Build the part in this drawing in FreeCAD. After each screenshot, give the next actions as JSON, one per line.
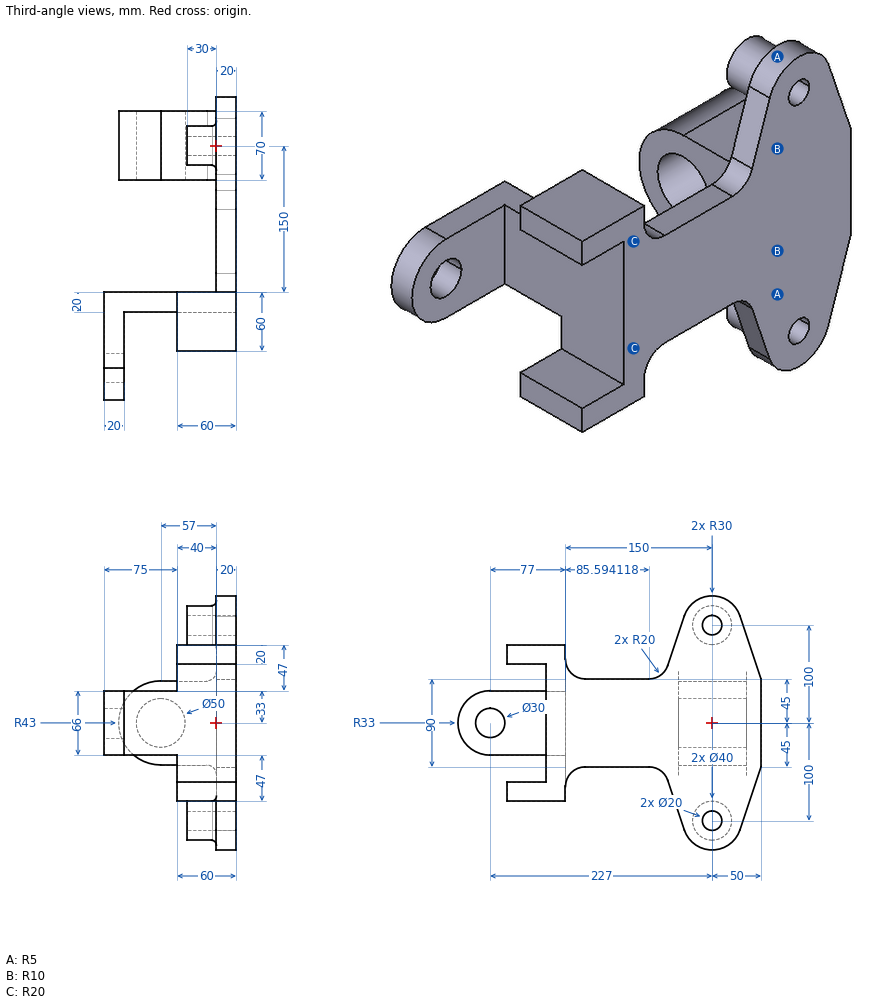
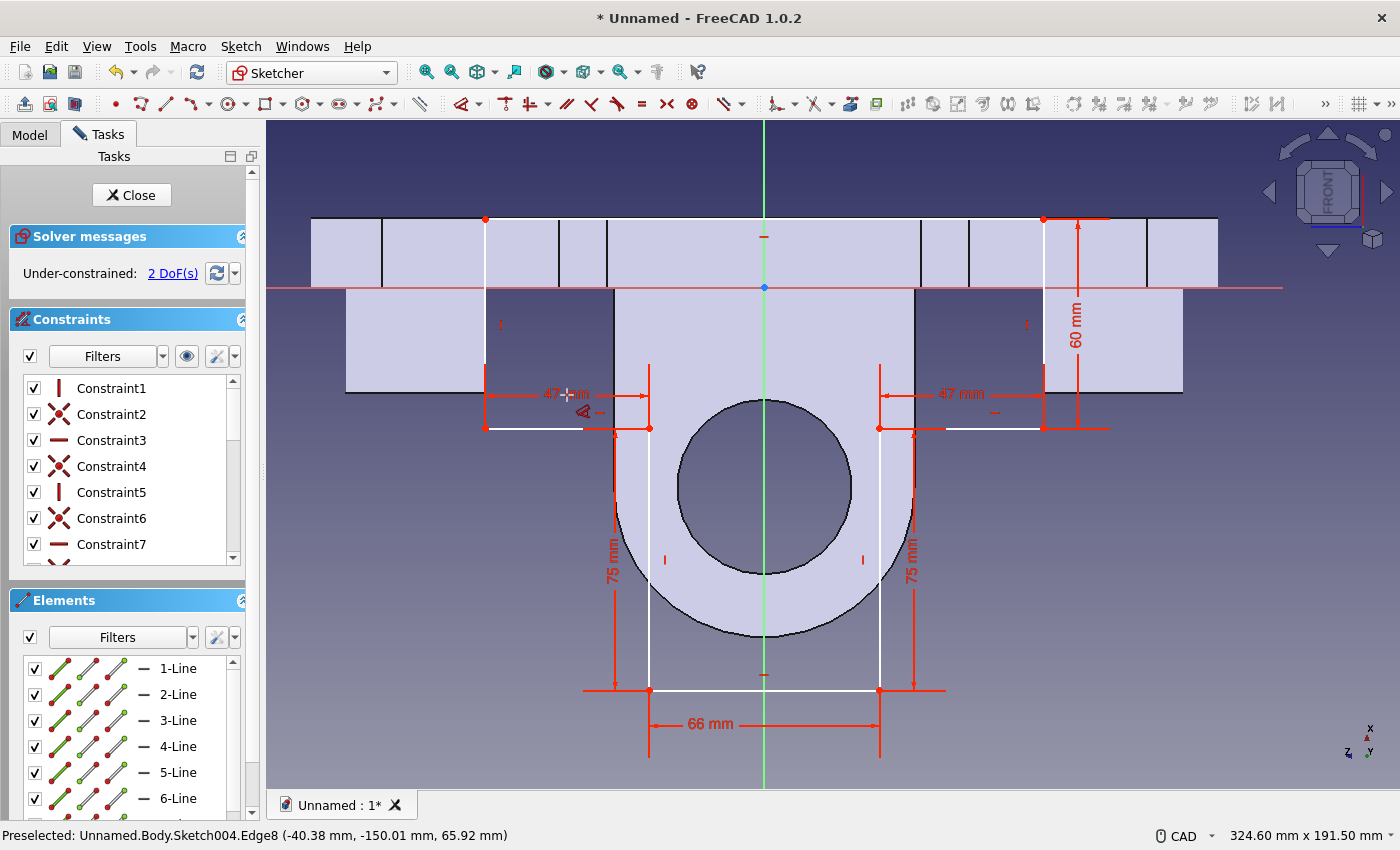
{"action": "left_click", "coordinate": [649, 429]}
{"action": "left_click", "coordinate": [707, 254]}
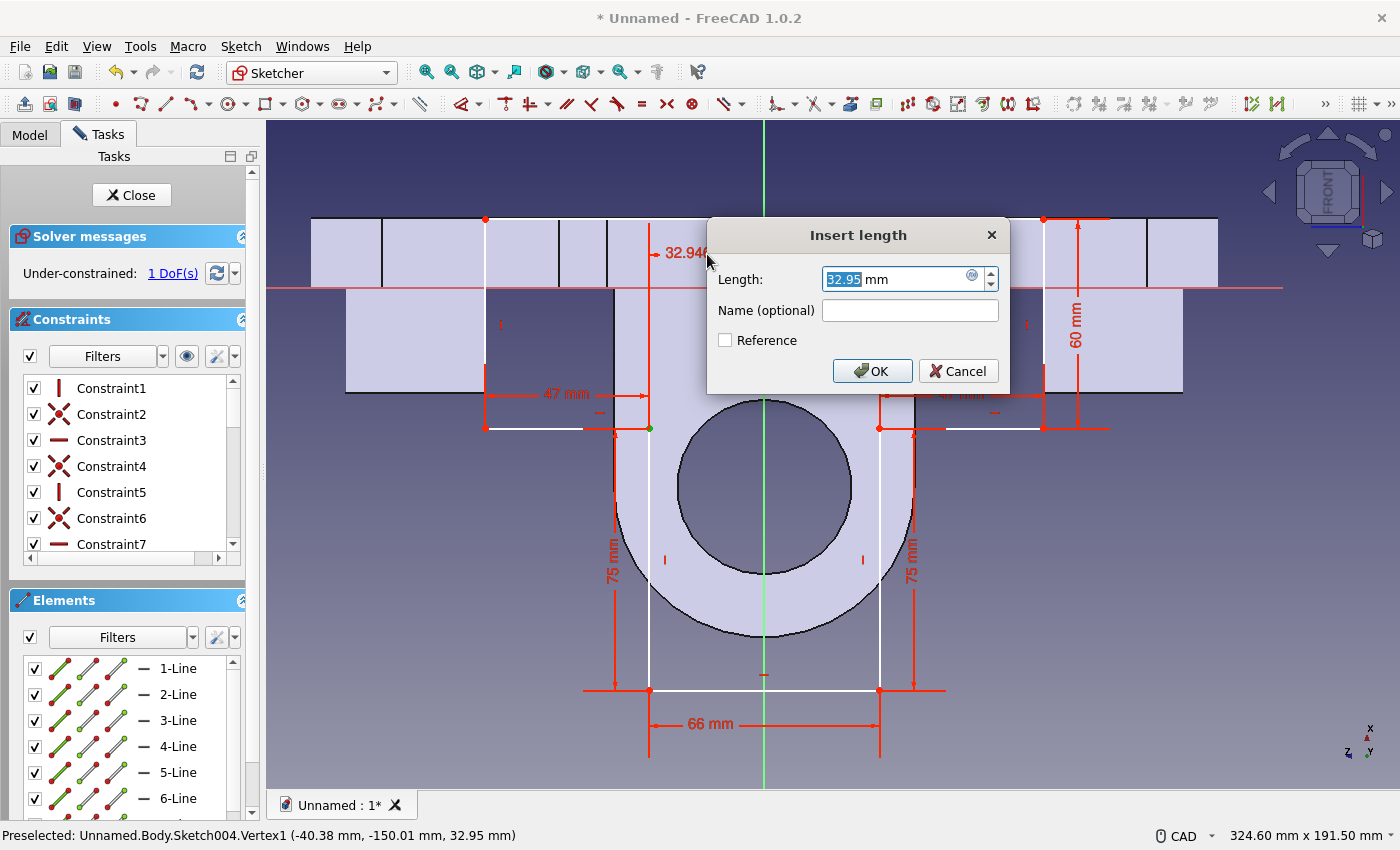
{"action": "type", "text": "33"}
{"action": "key", "text": "Return"}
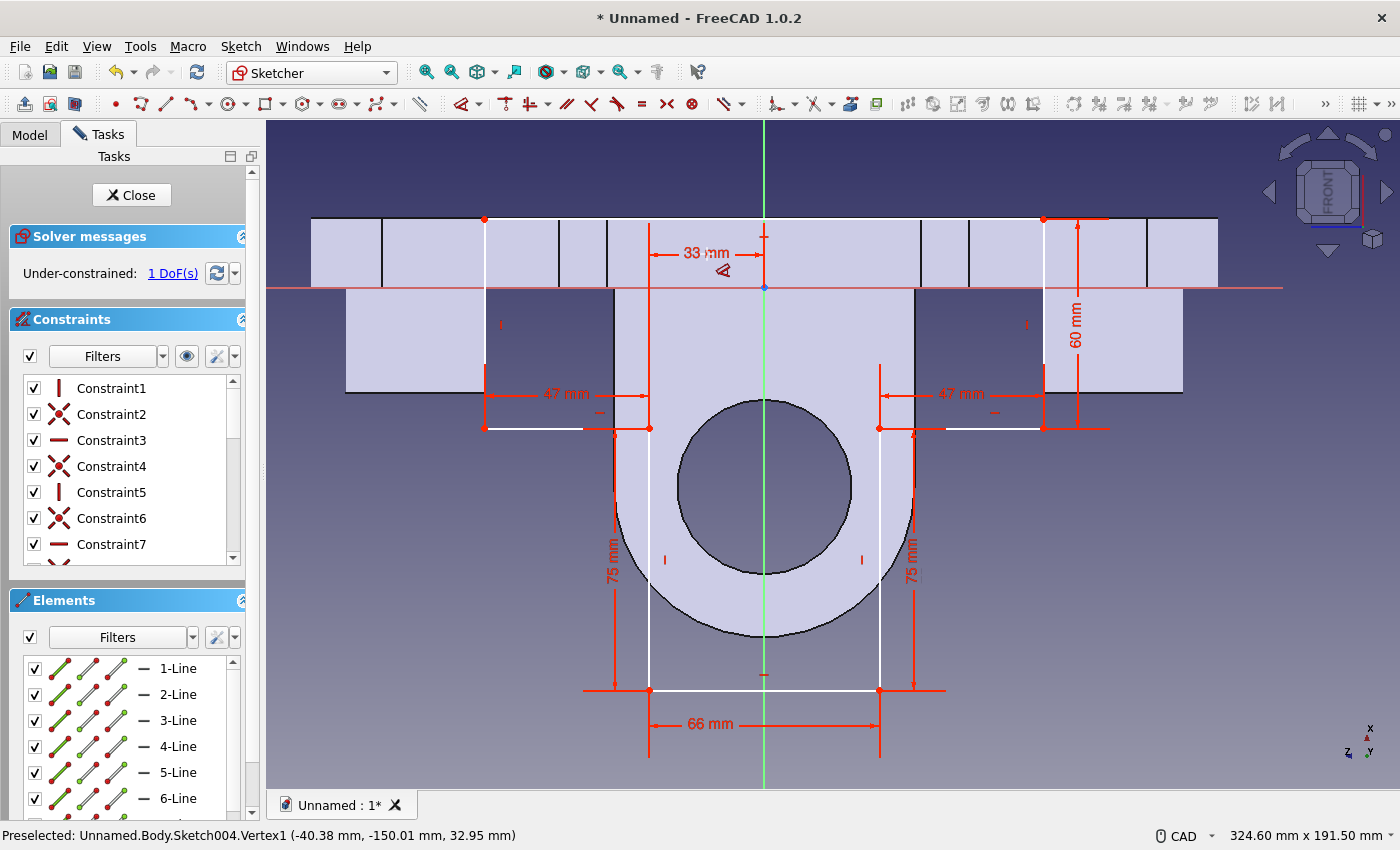
{"action": "left_click", "coordinate": [649, 429]}
{"action": "left_click", "coordinate": [615, 358]}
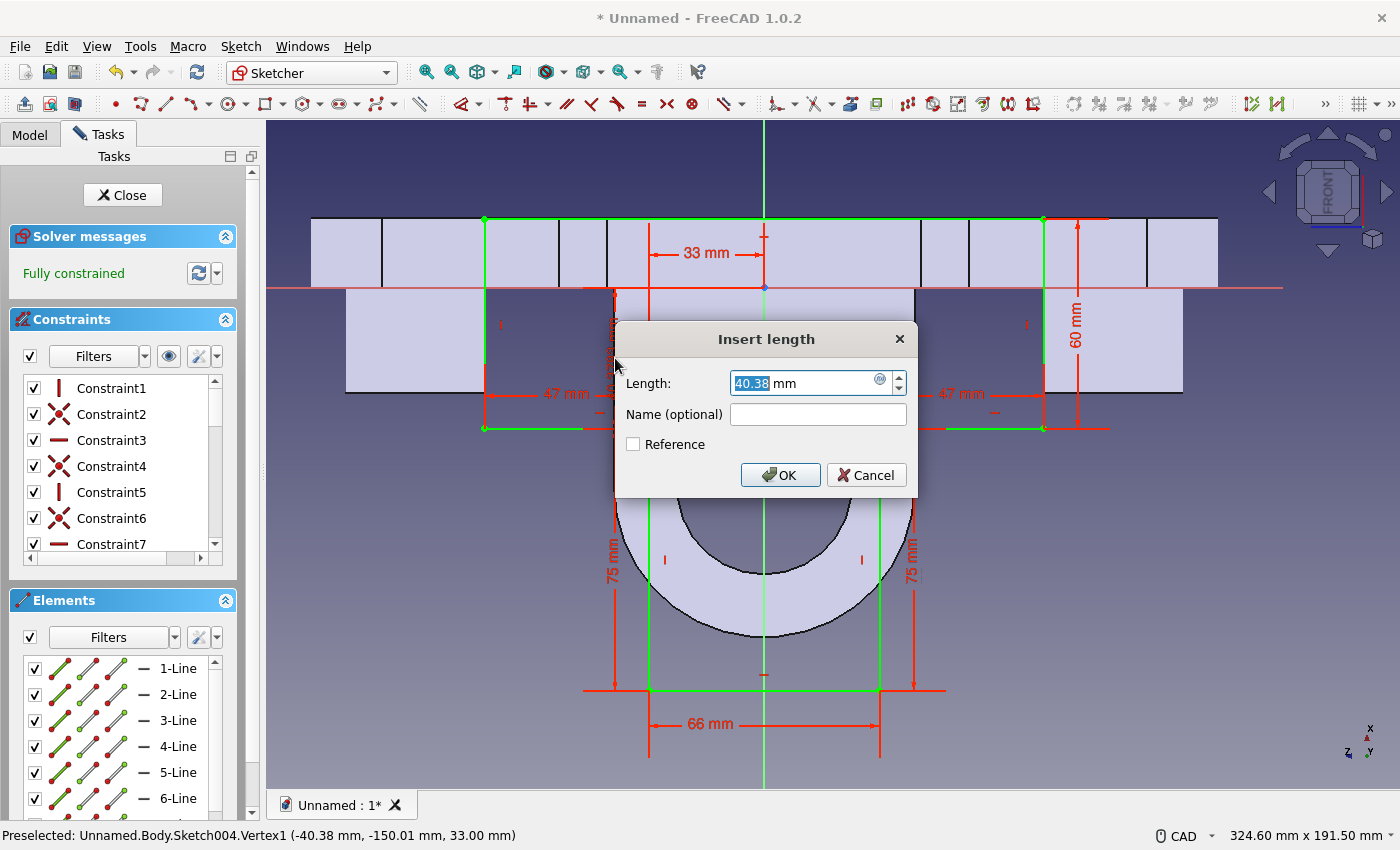
{"action": "type", "text": "40"}
{"action": "key", "text": "Return"}
{"action": "key", "text": "Escape"}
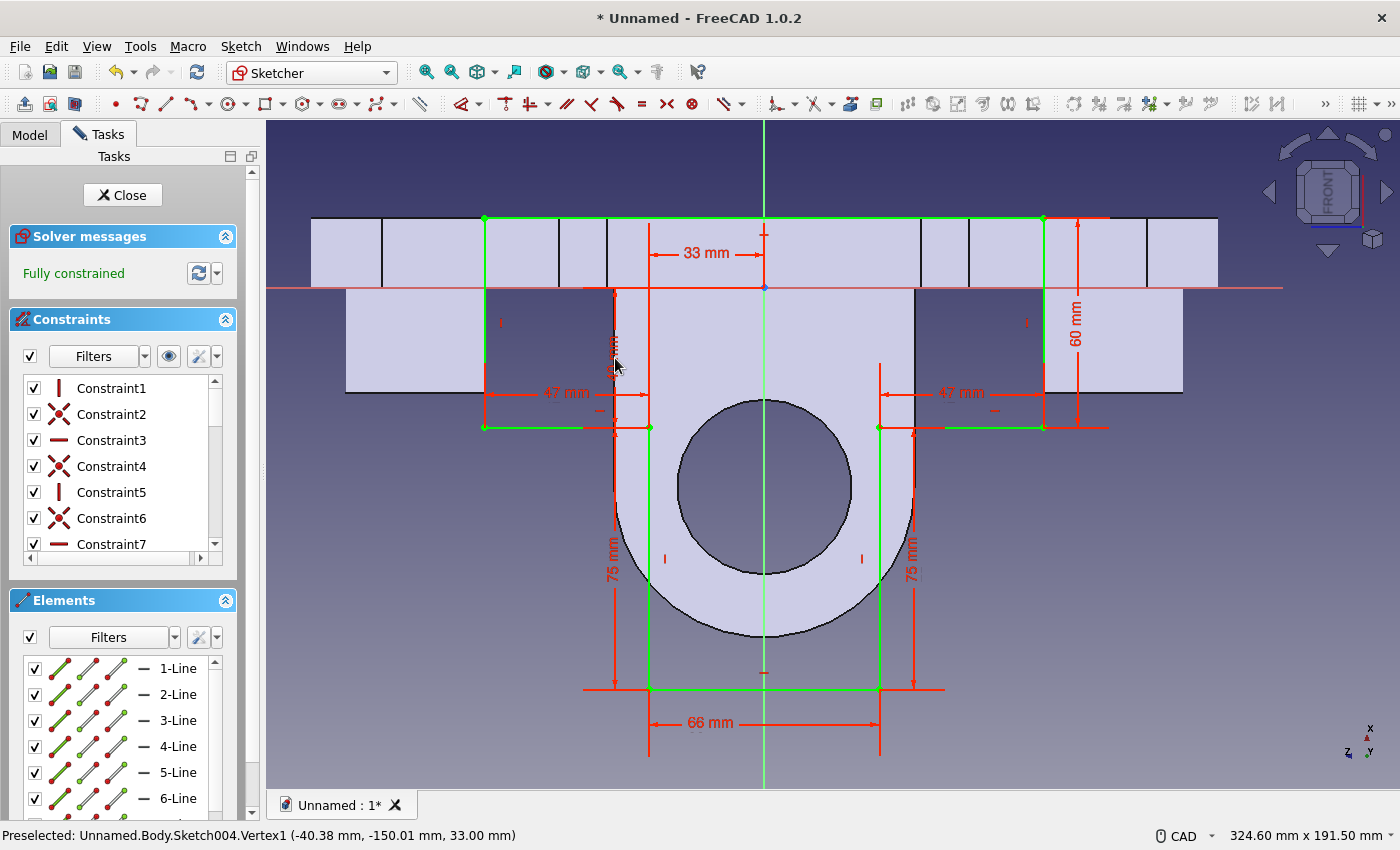
{"action": "left_click", "coordinate": [123, 195]}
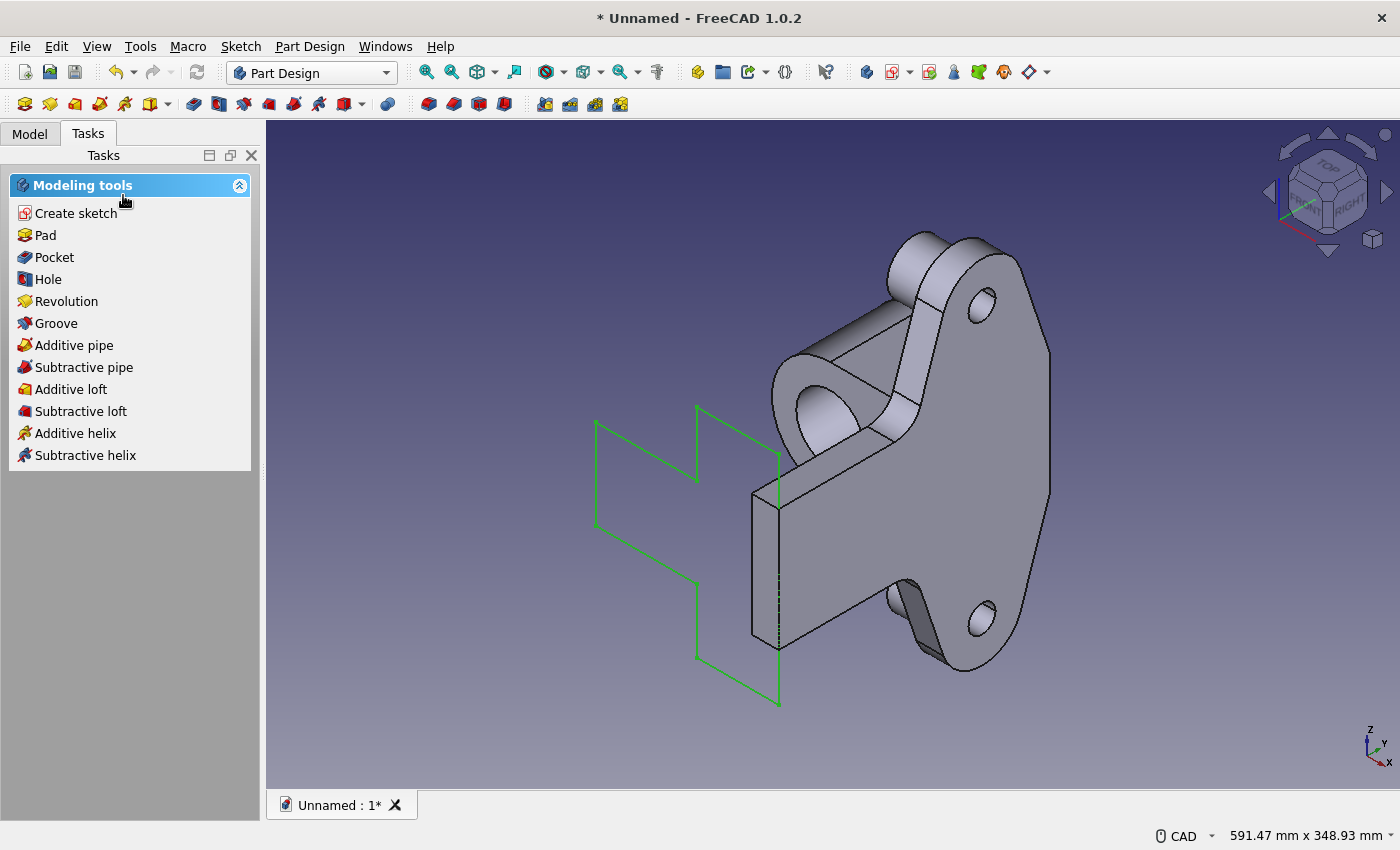
{"action": "left_click", "coordinate": [25, 104]}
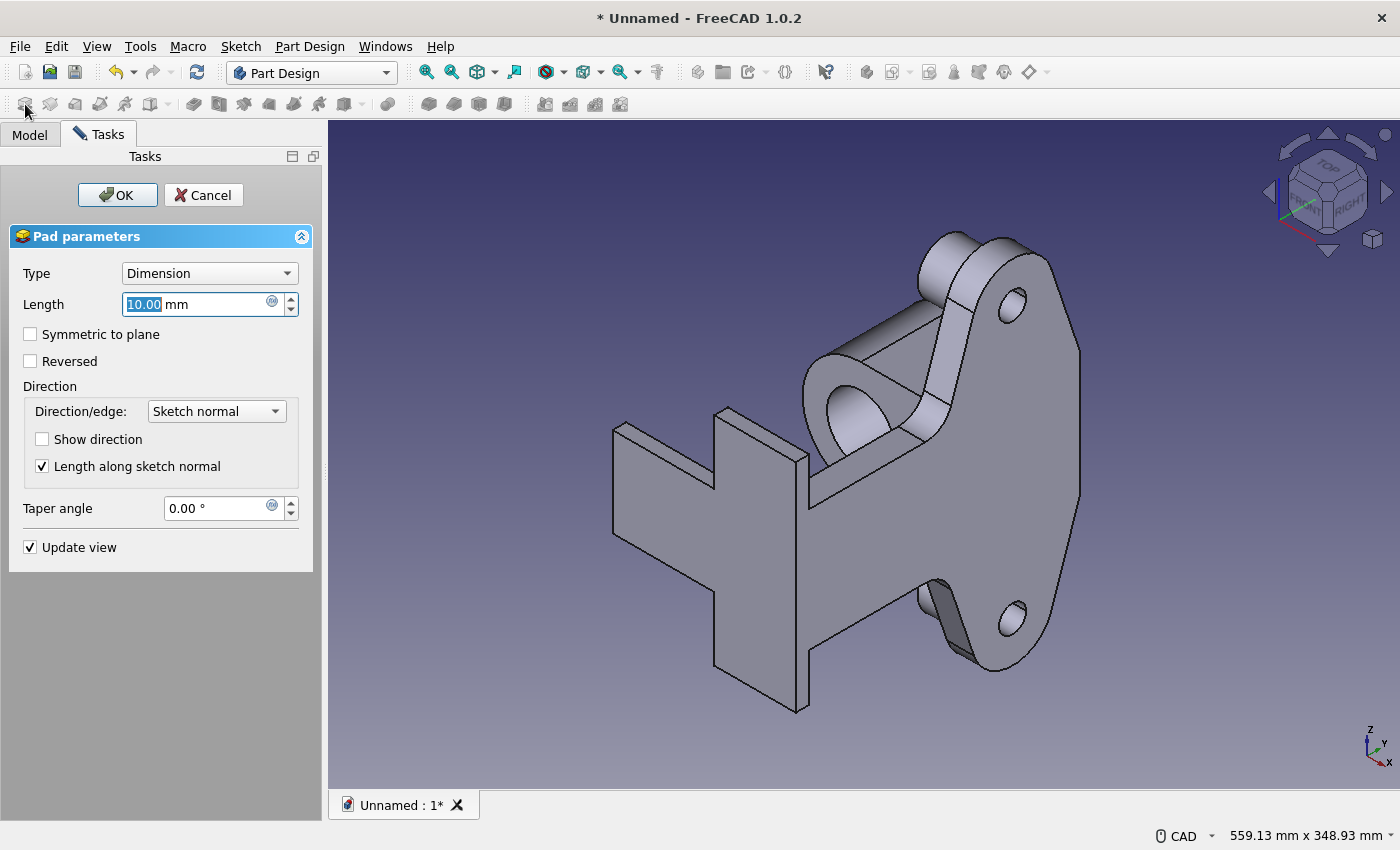
{"action": "type", "text": "20"}
{"action": "key", "text": "Tab"}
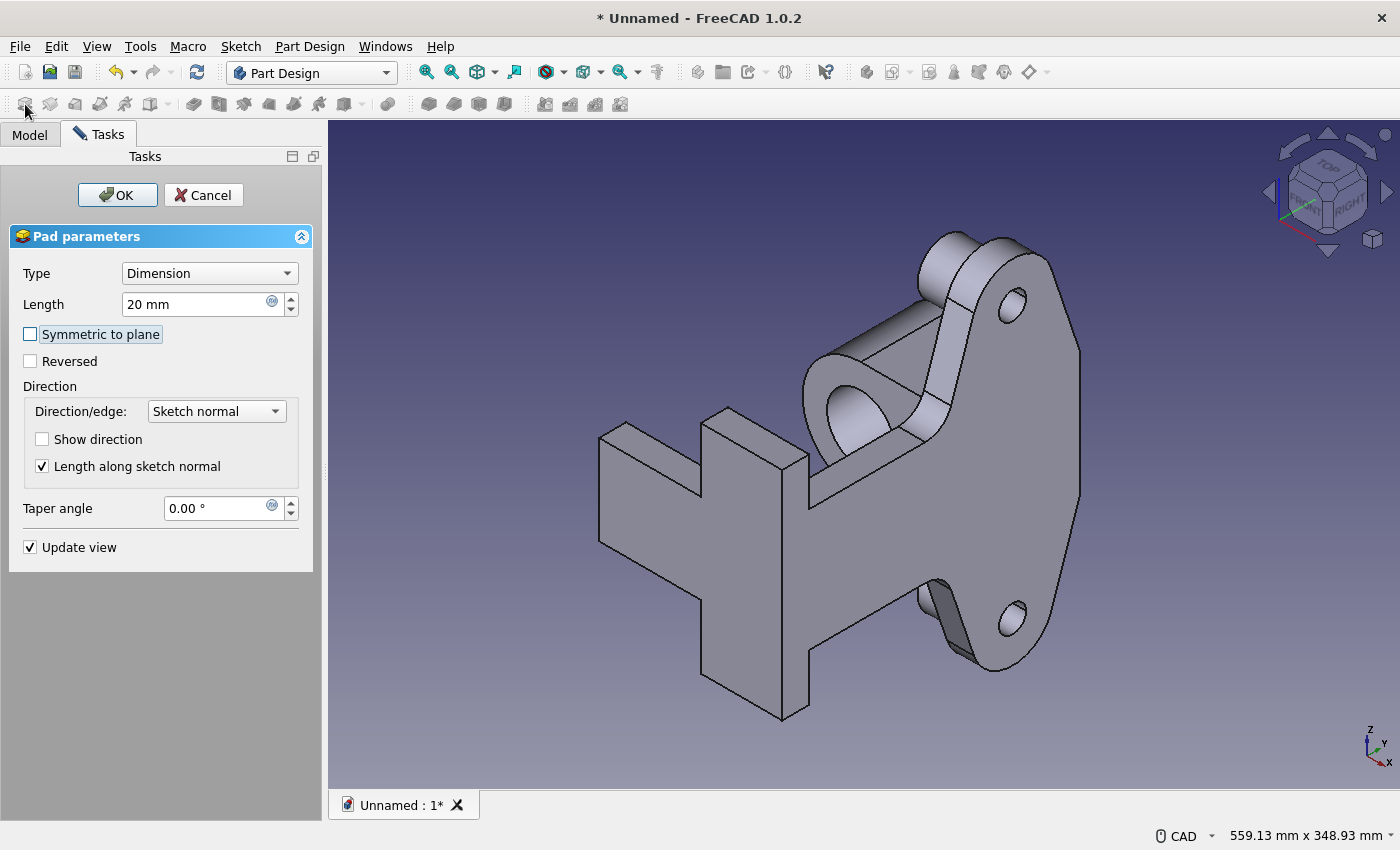
{"action": "left_click", "coordinate": [118, 195]}